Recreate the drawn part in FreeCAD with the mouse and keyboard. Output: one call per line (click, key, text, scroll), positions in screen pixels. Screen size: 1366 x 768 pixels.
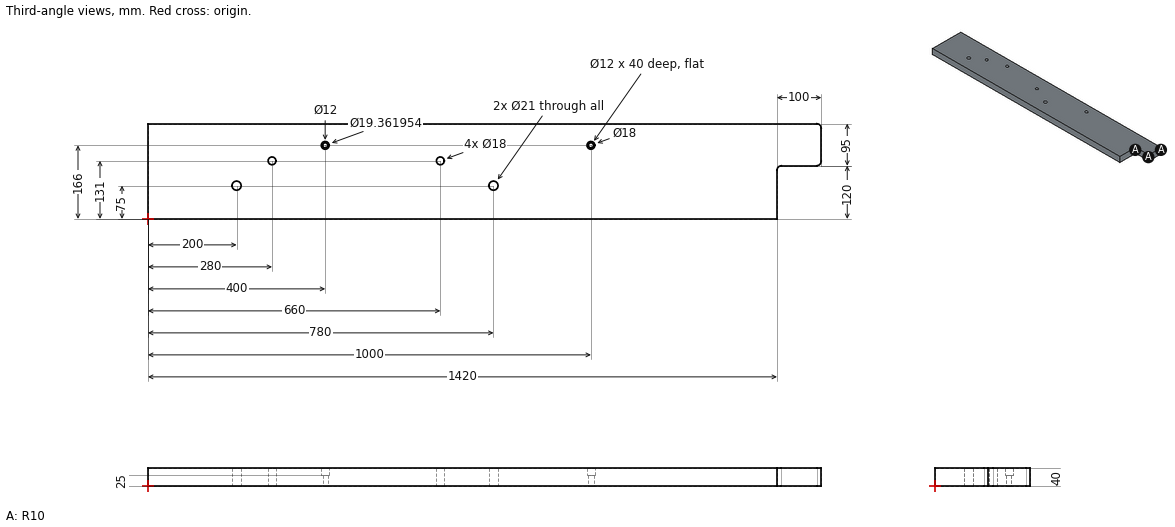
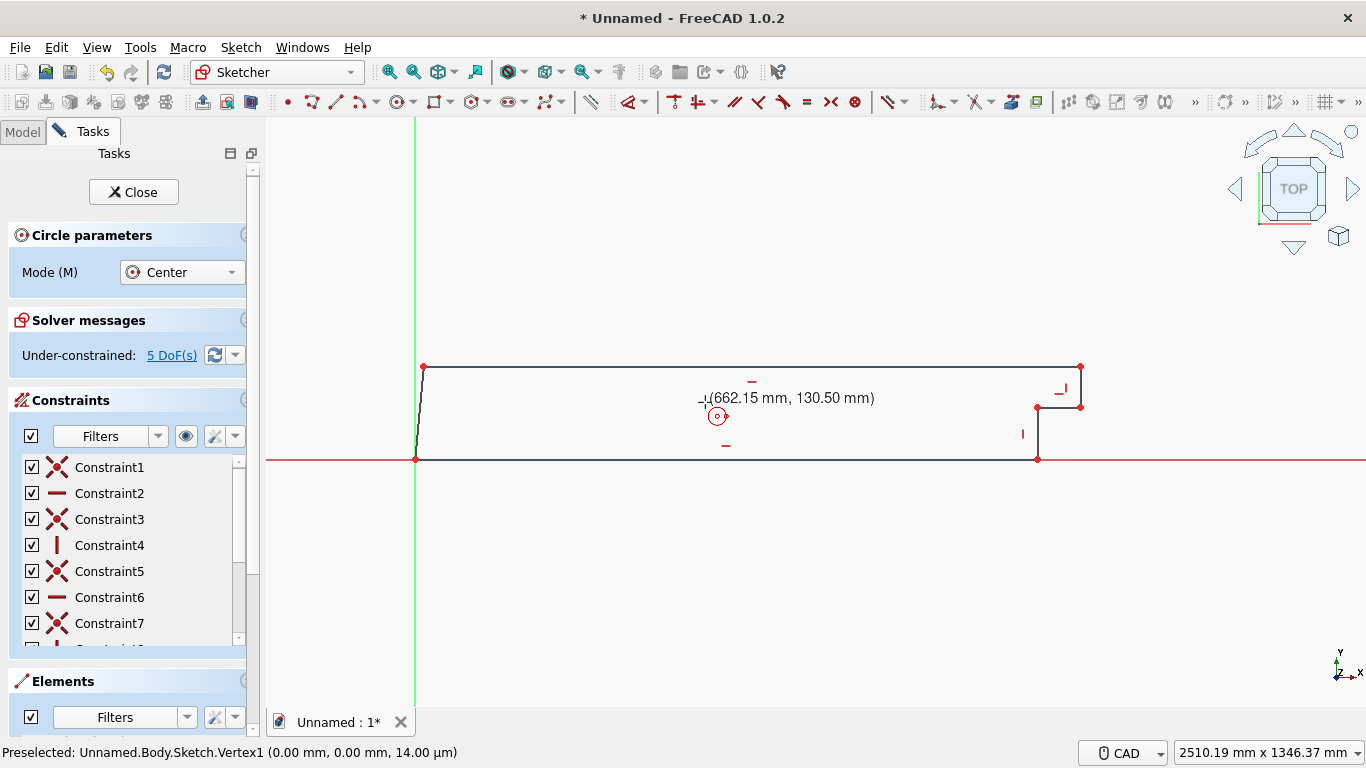
click(704, 402)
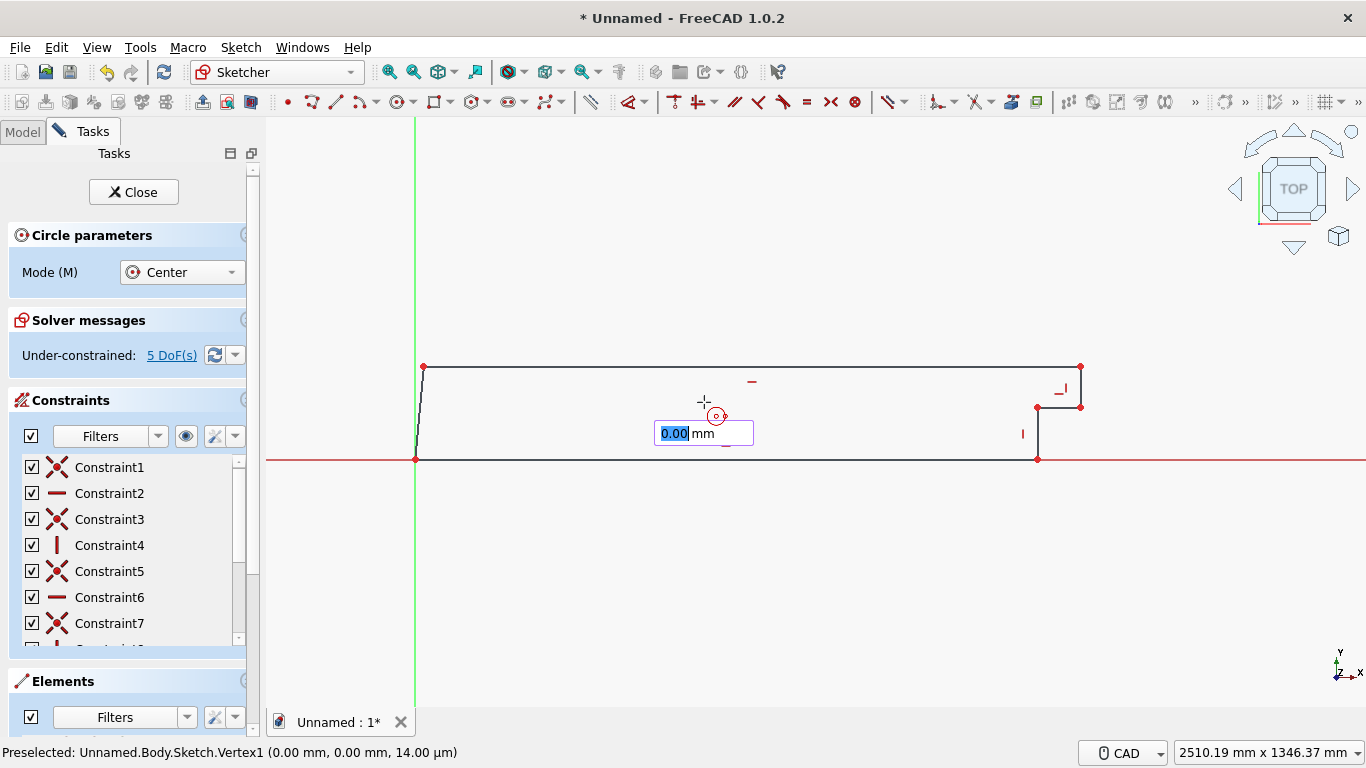
scroll(707, 400, up, 7)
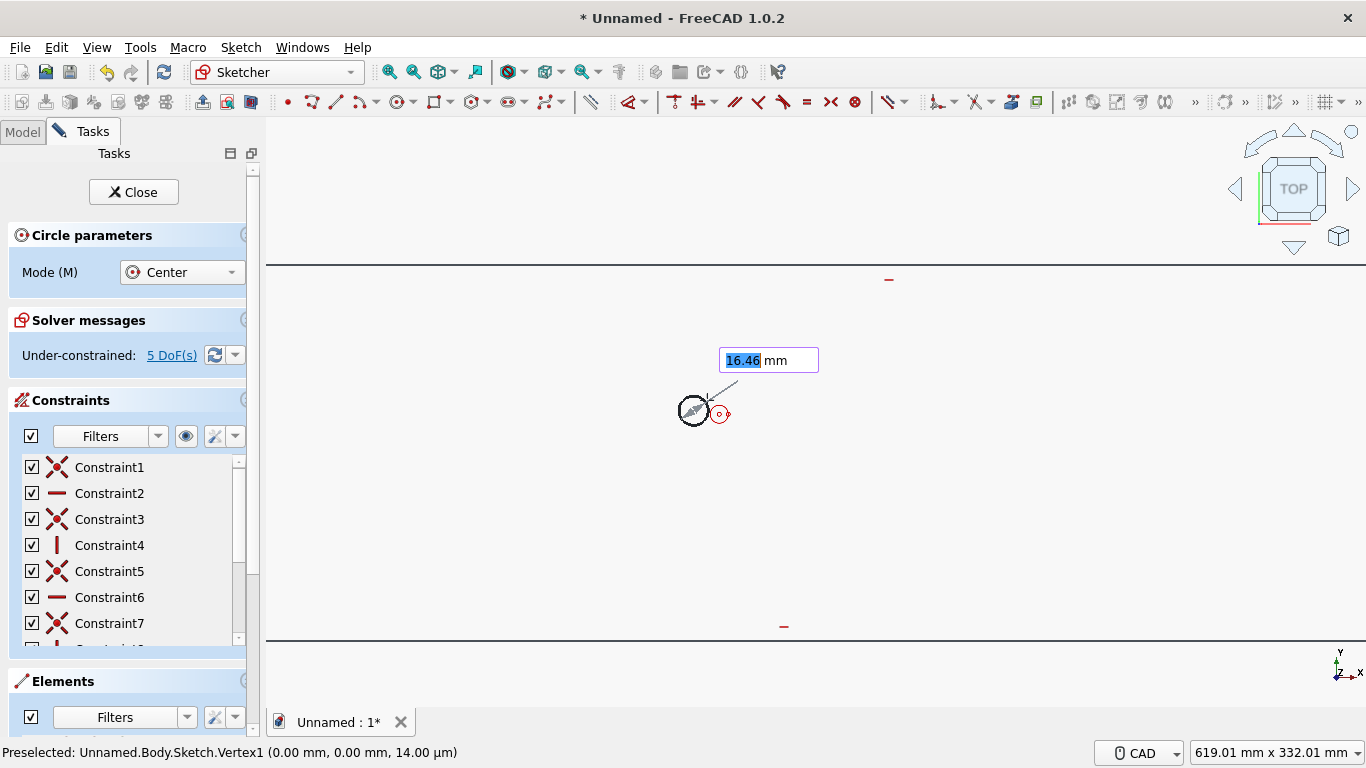
click(706, 397)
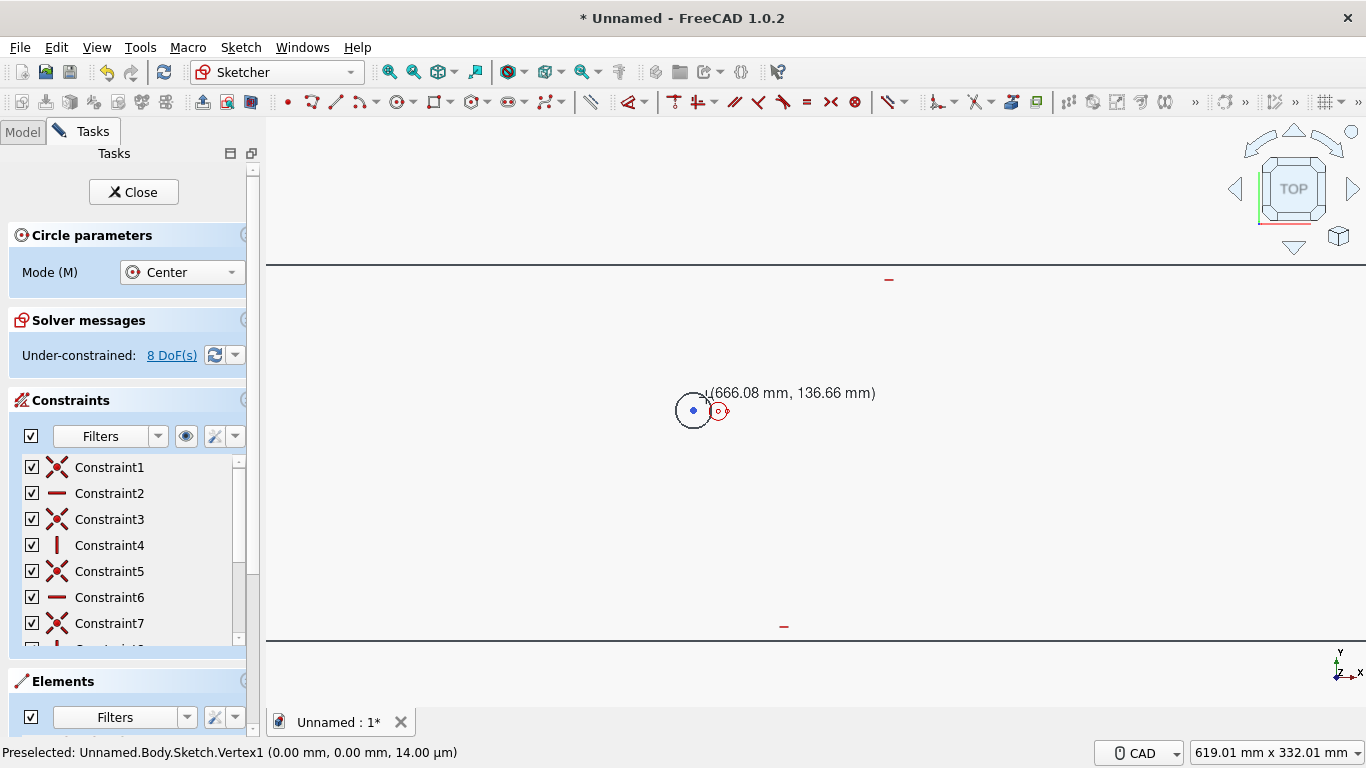
scroll(706, 400, down, 7)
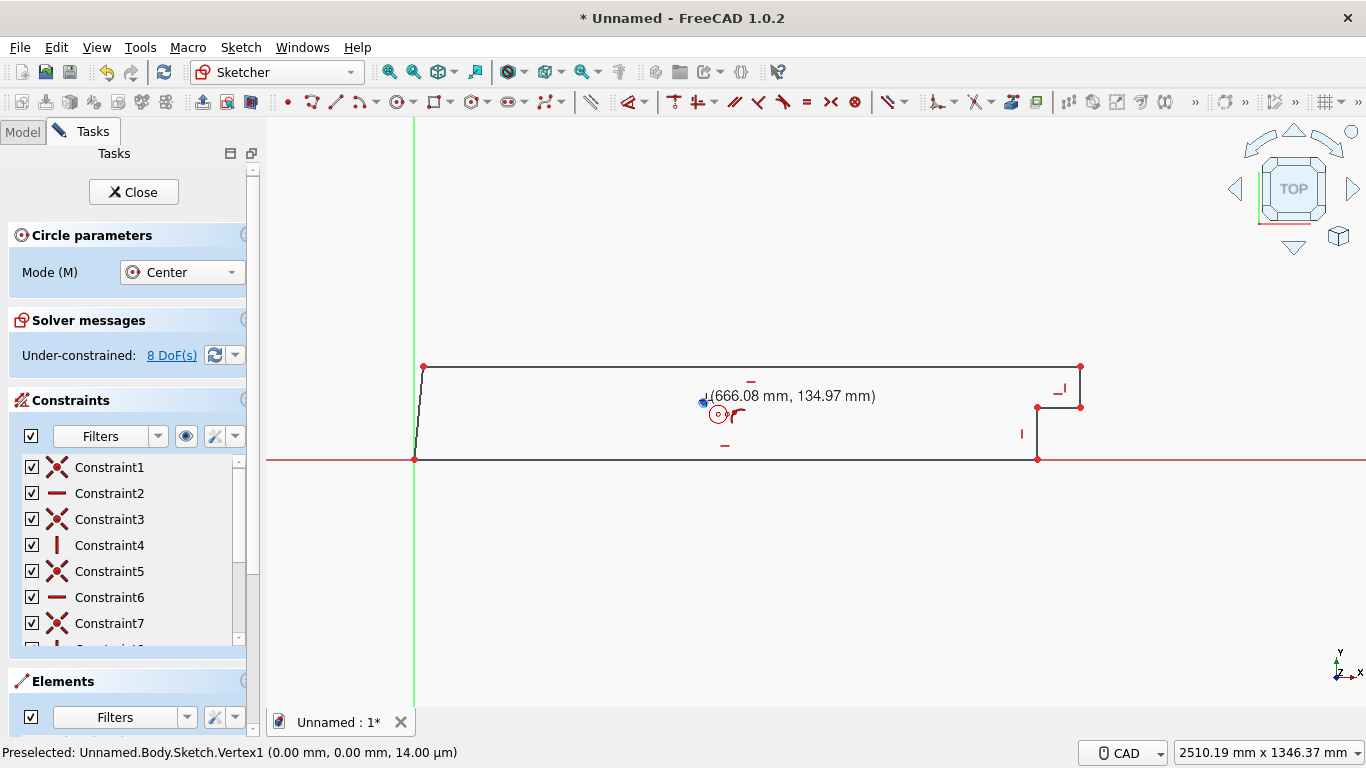
scroll(537, 402, up, 9)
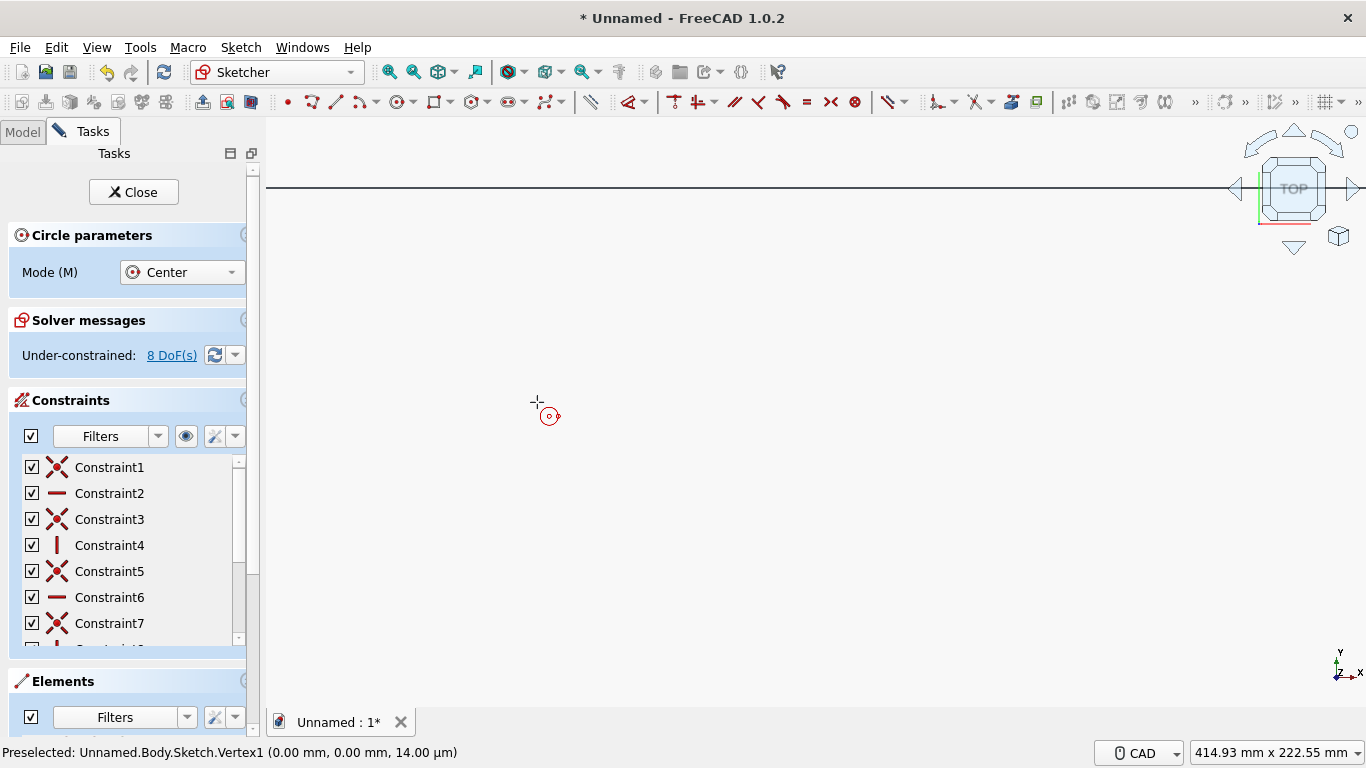
scroll(537, 402, down, 9)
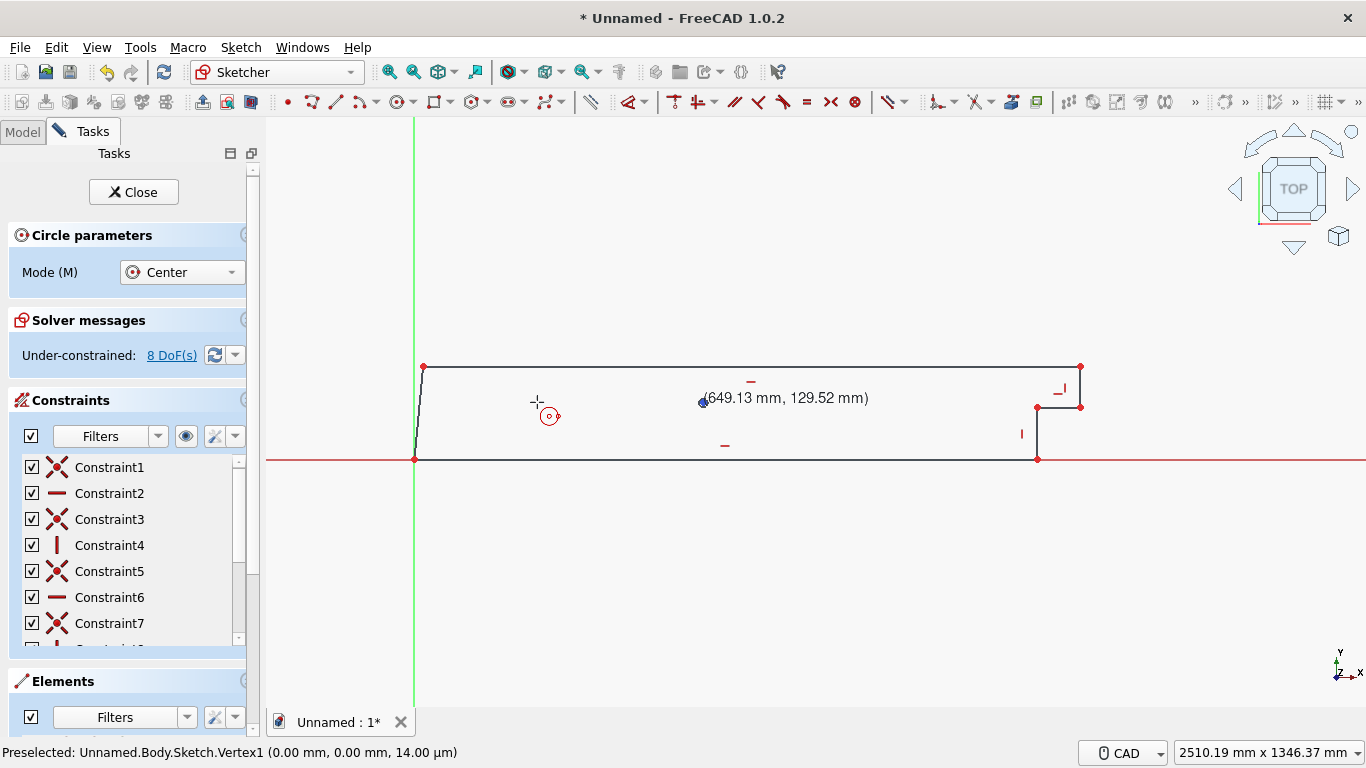
click(537, 402)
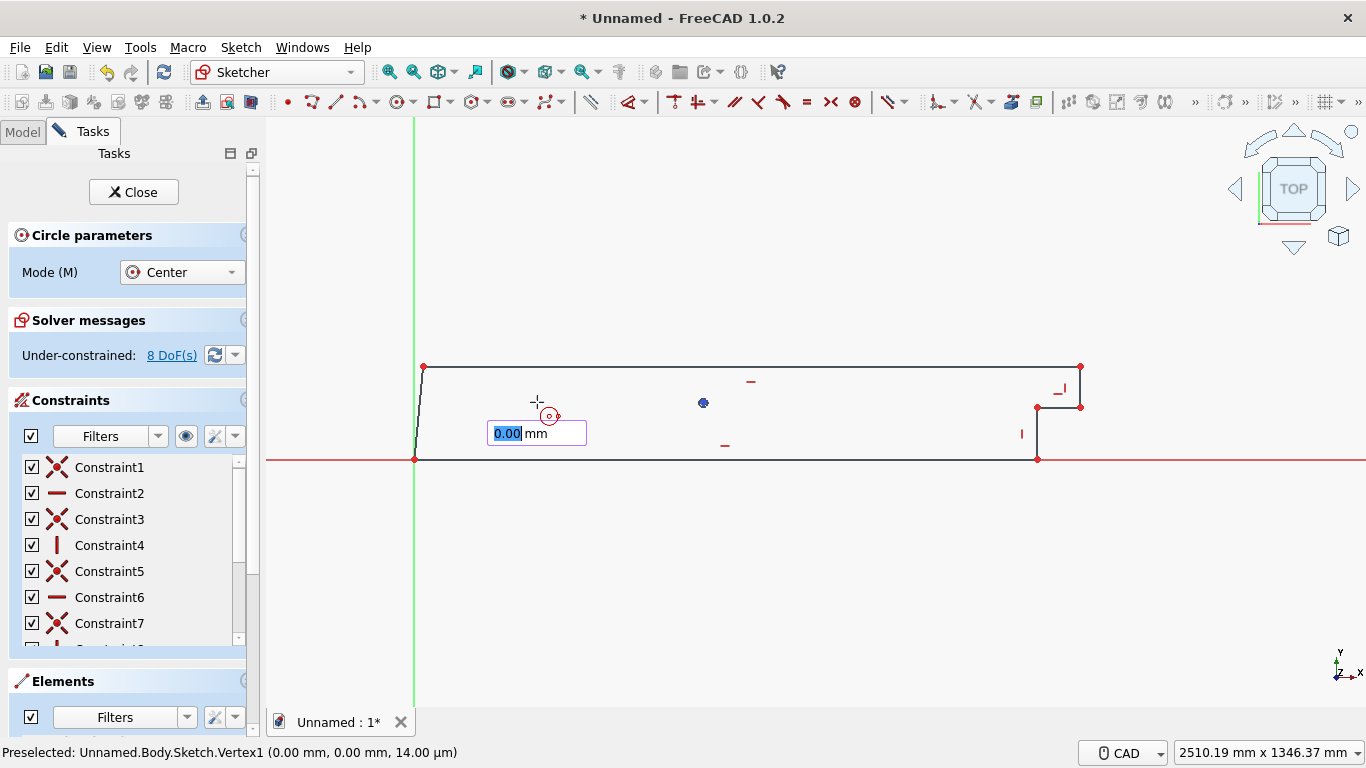
scroll(540, 400, up, 7)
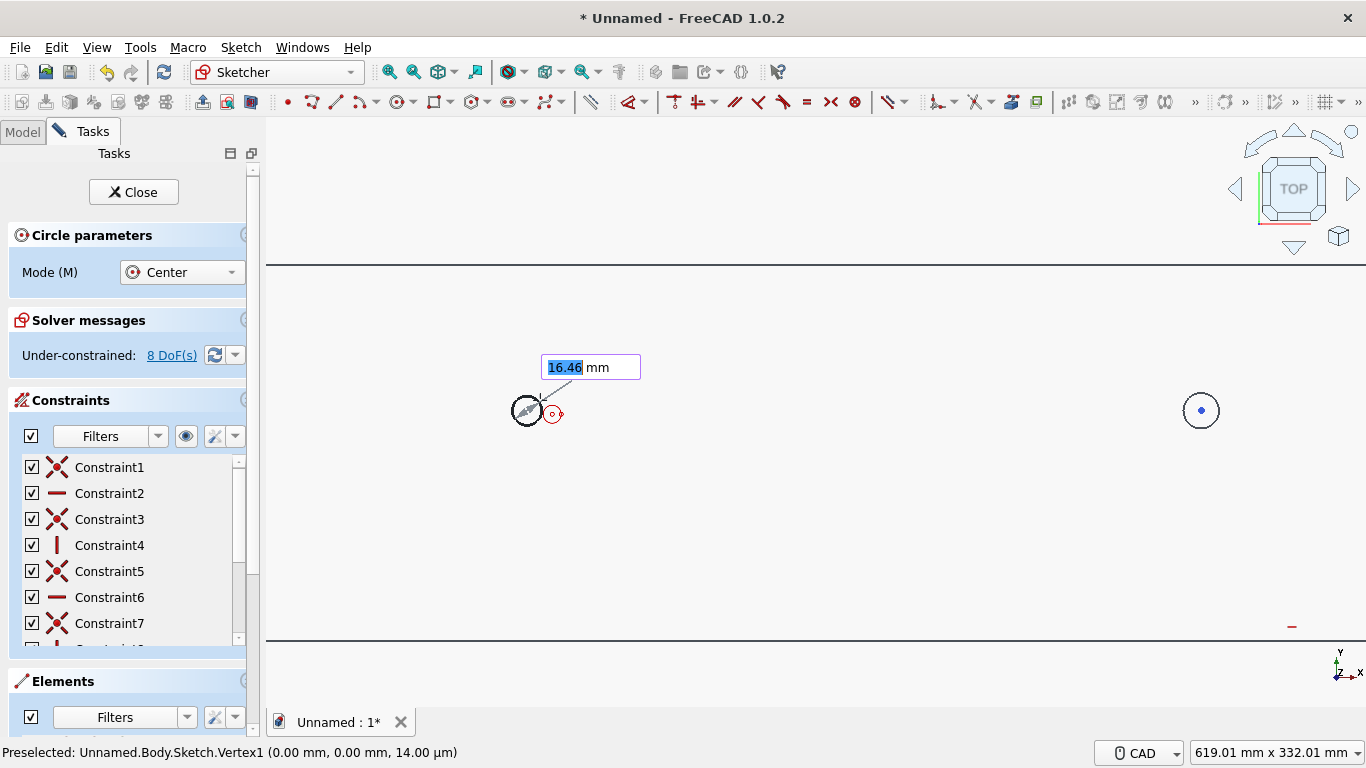
click(539, 397)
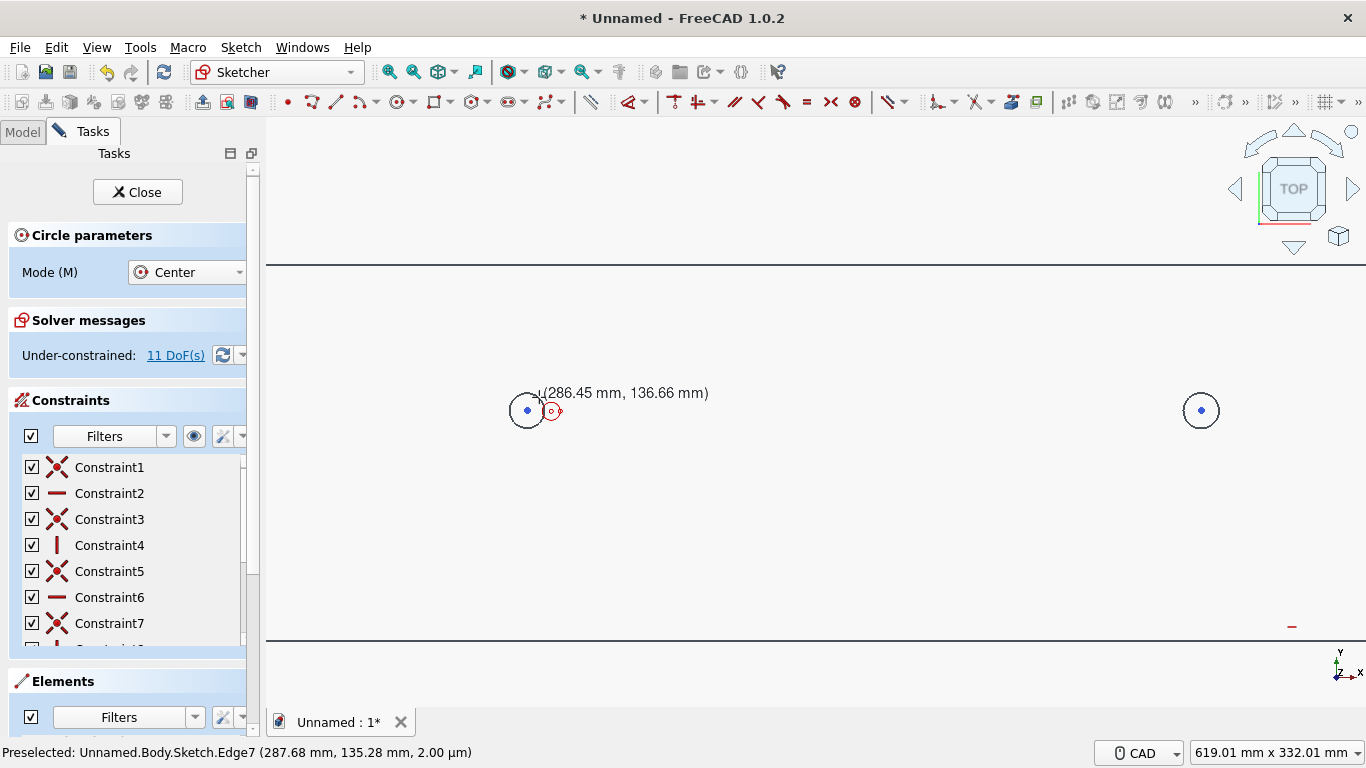
scroll(540, 400, down, 7)